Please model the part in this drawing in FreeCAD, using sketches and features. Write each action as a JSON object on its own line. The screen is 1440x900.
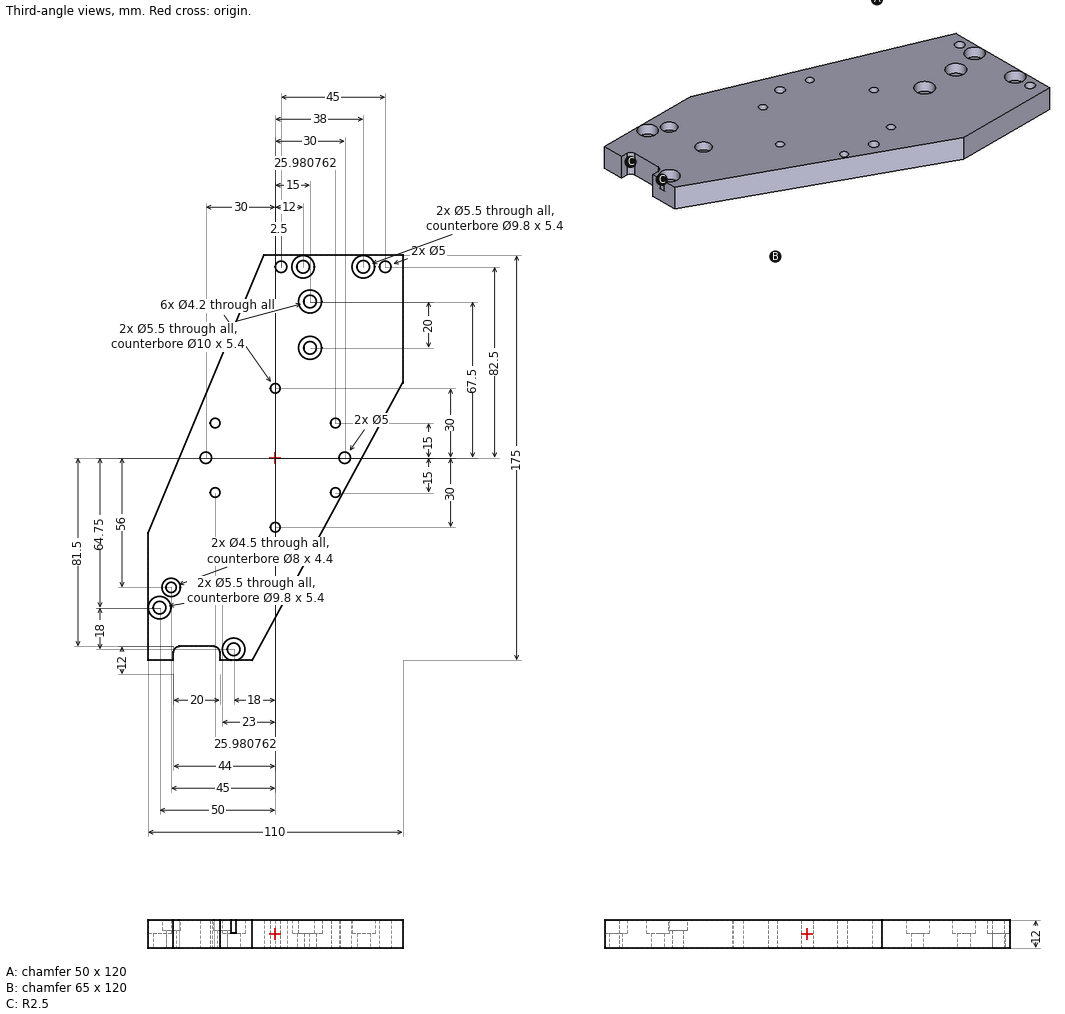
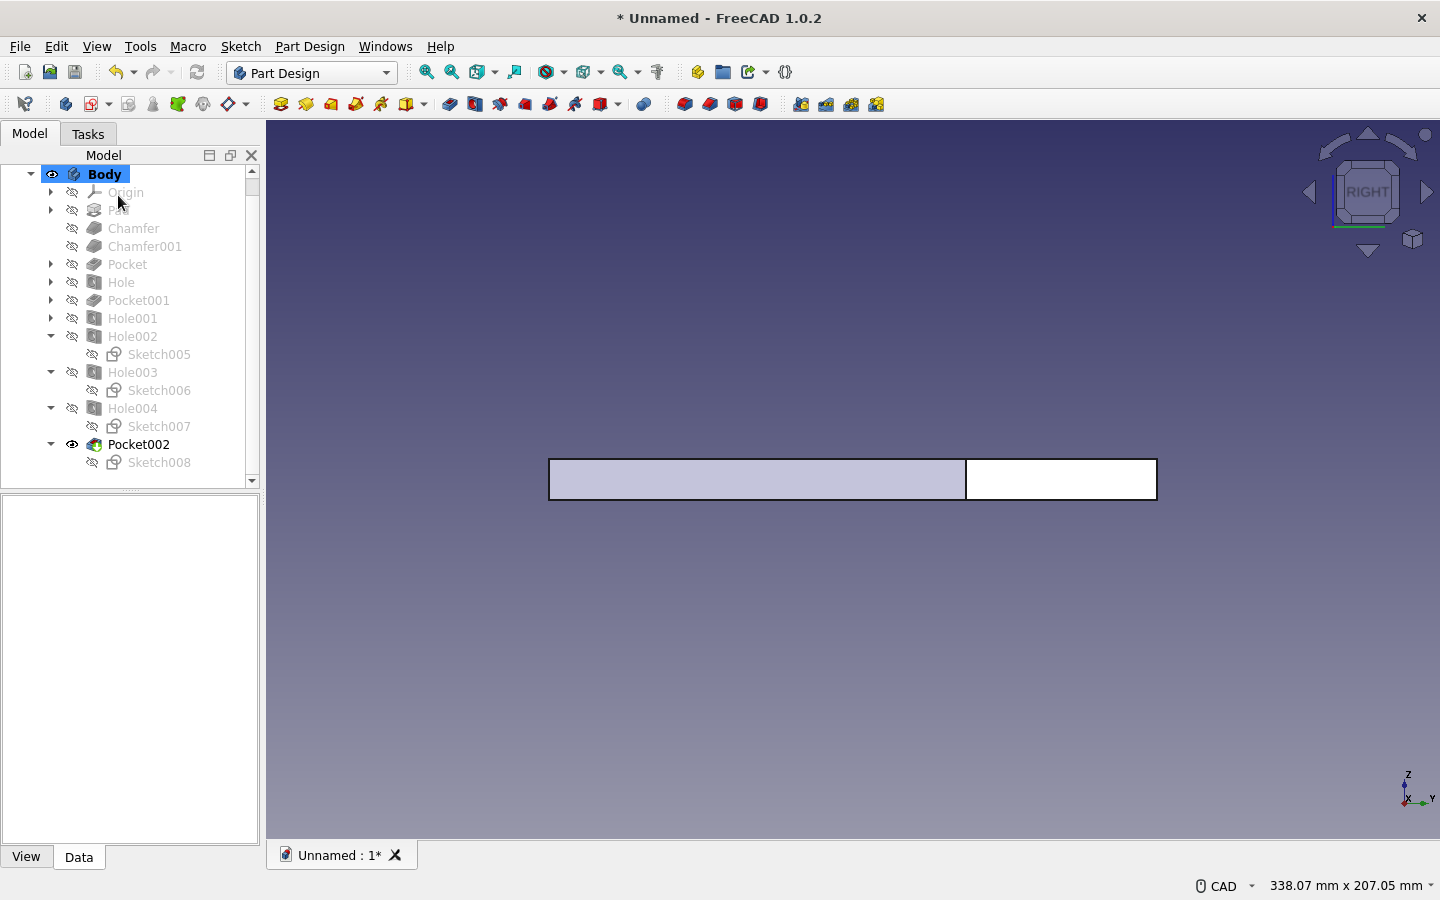
{"action": "key", "text": "5"}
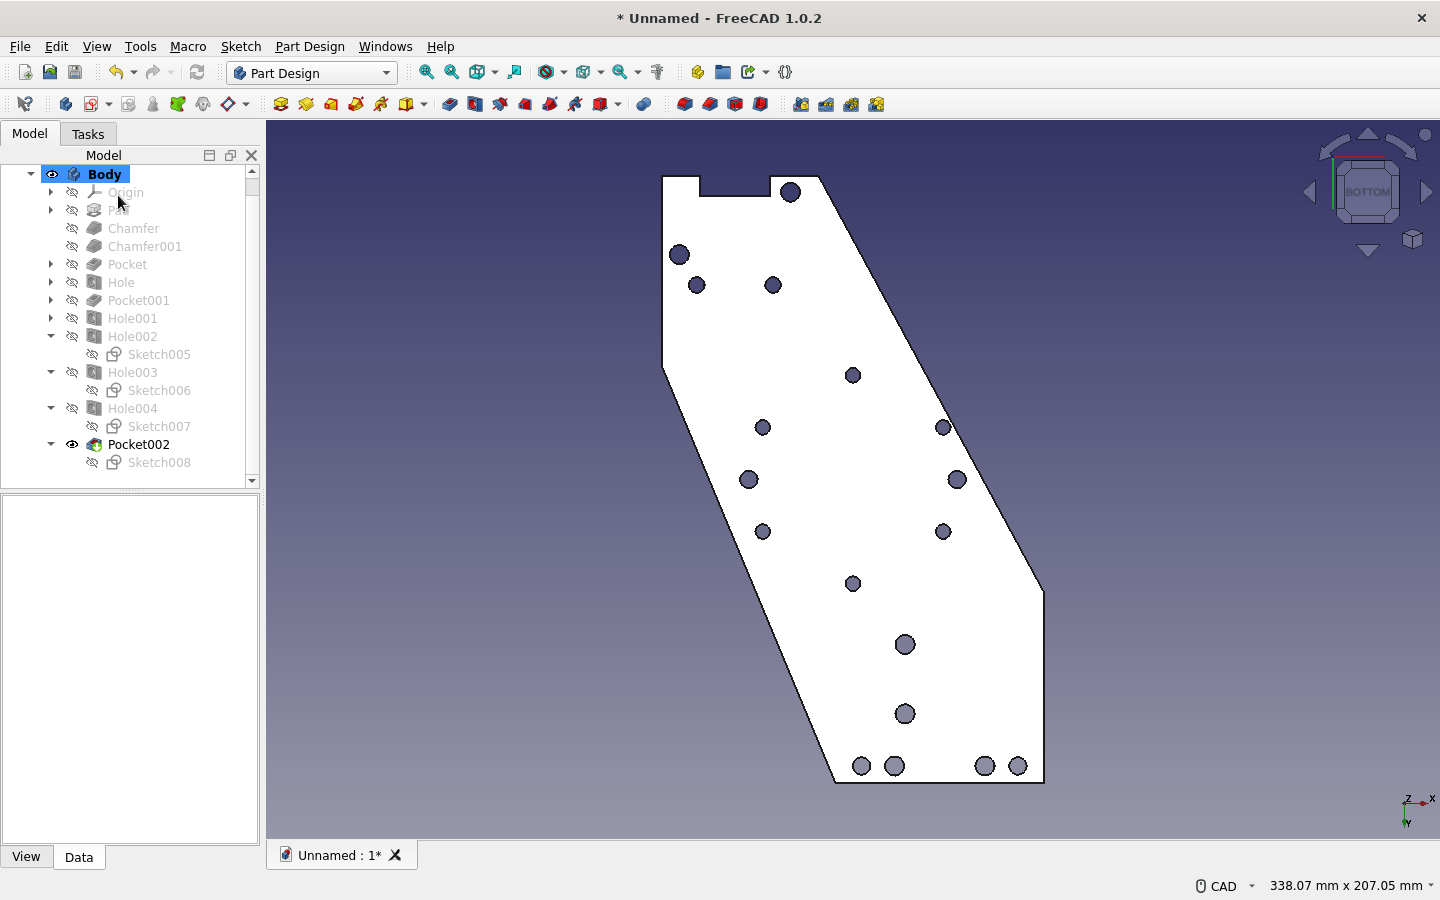
{"action": "key", "text": "4"}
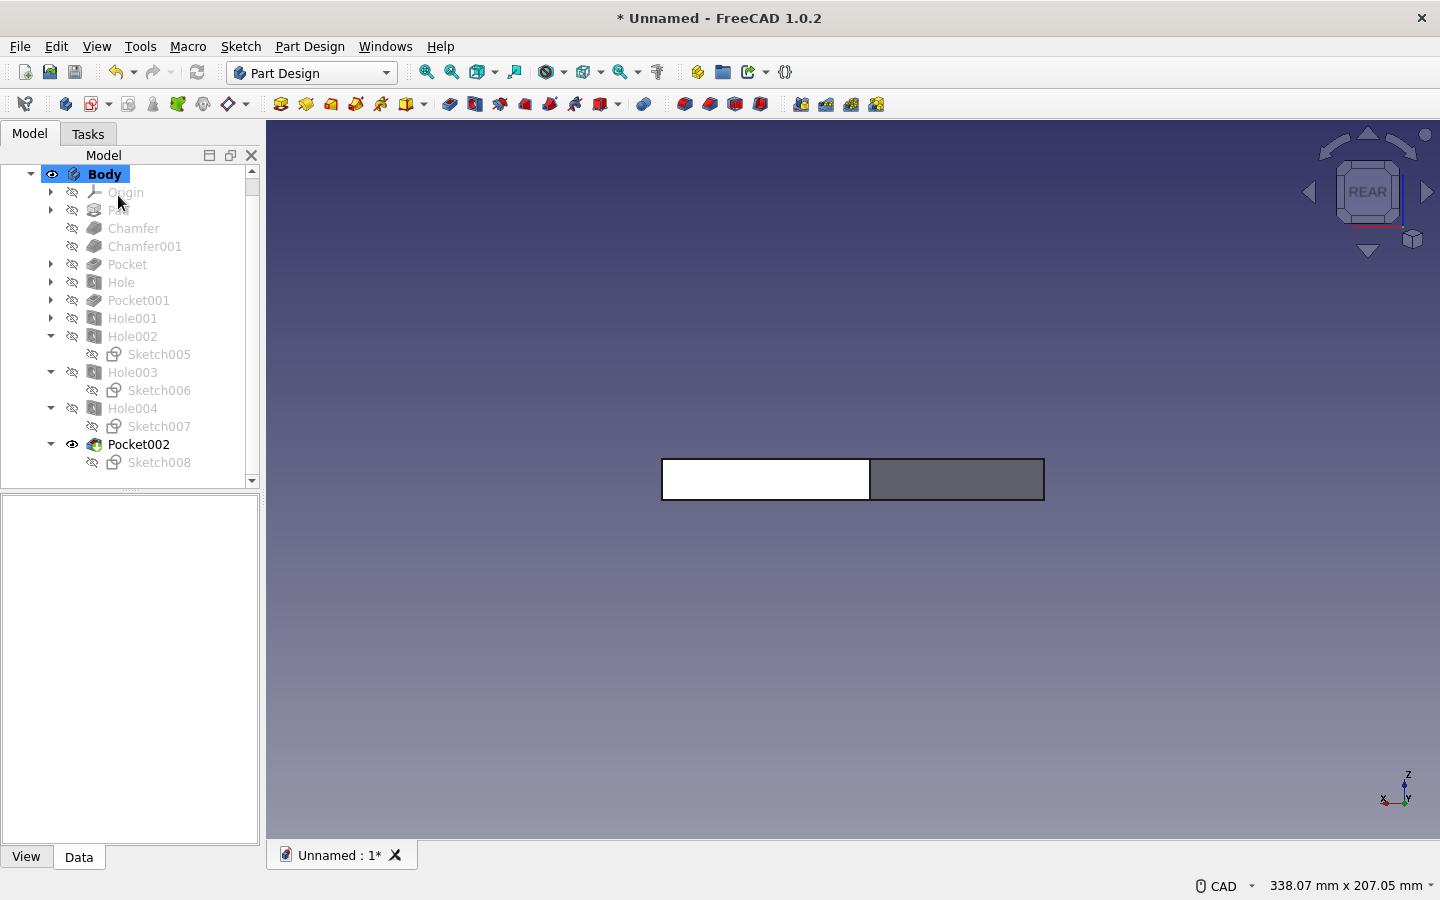
{"action": "key", "text": "v f"}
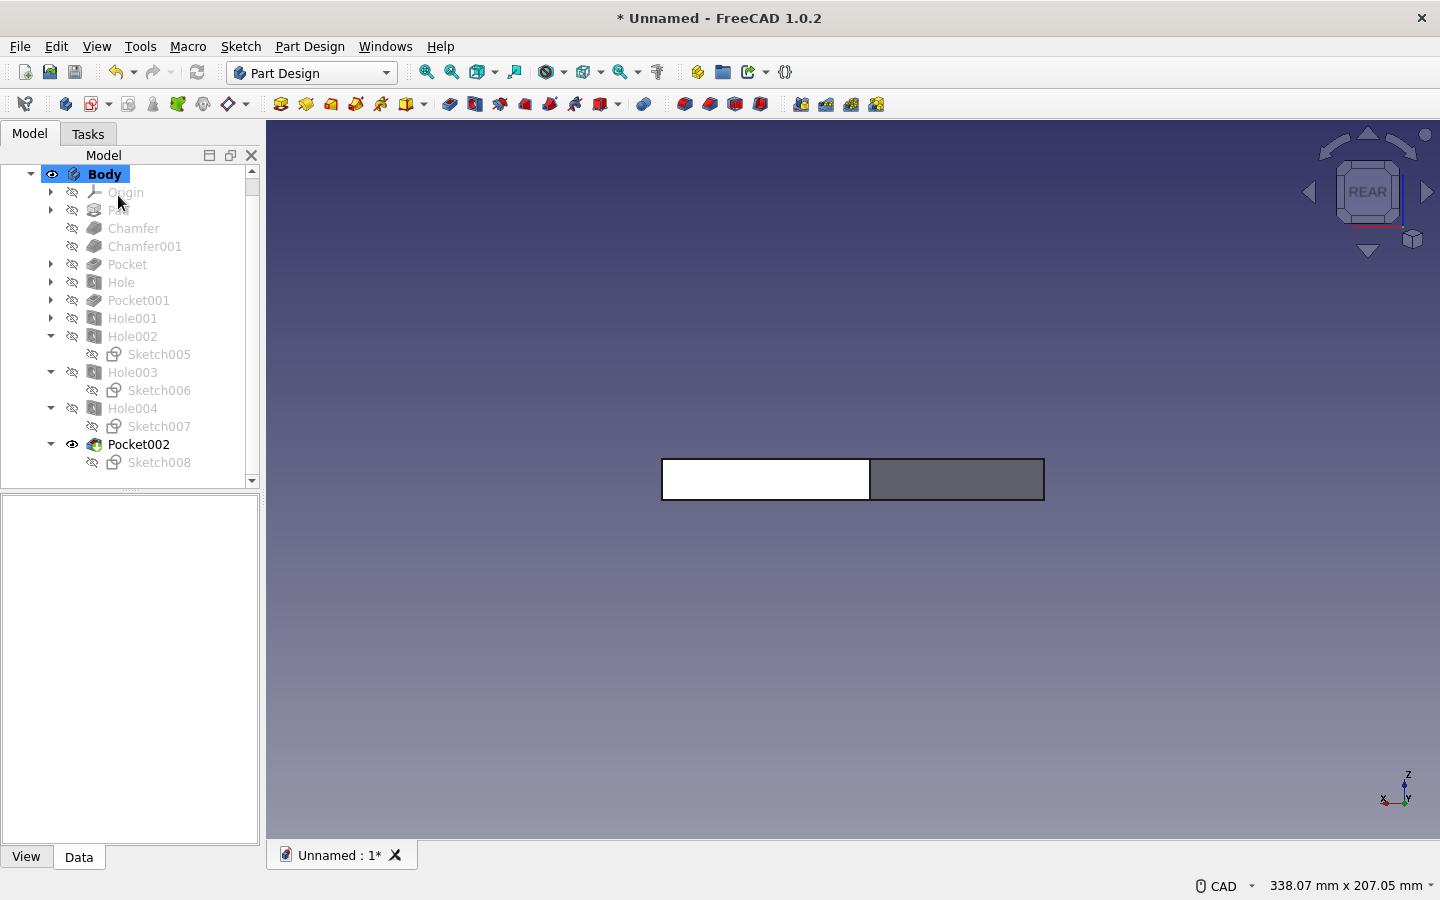
{"action": "key", "text": "6"}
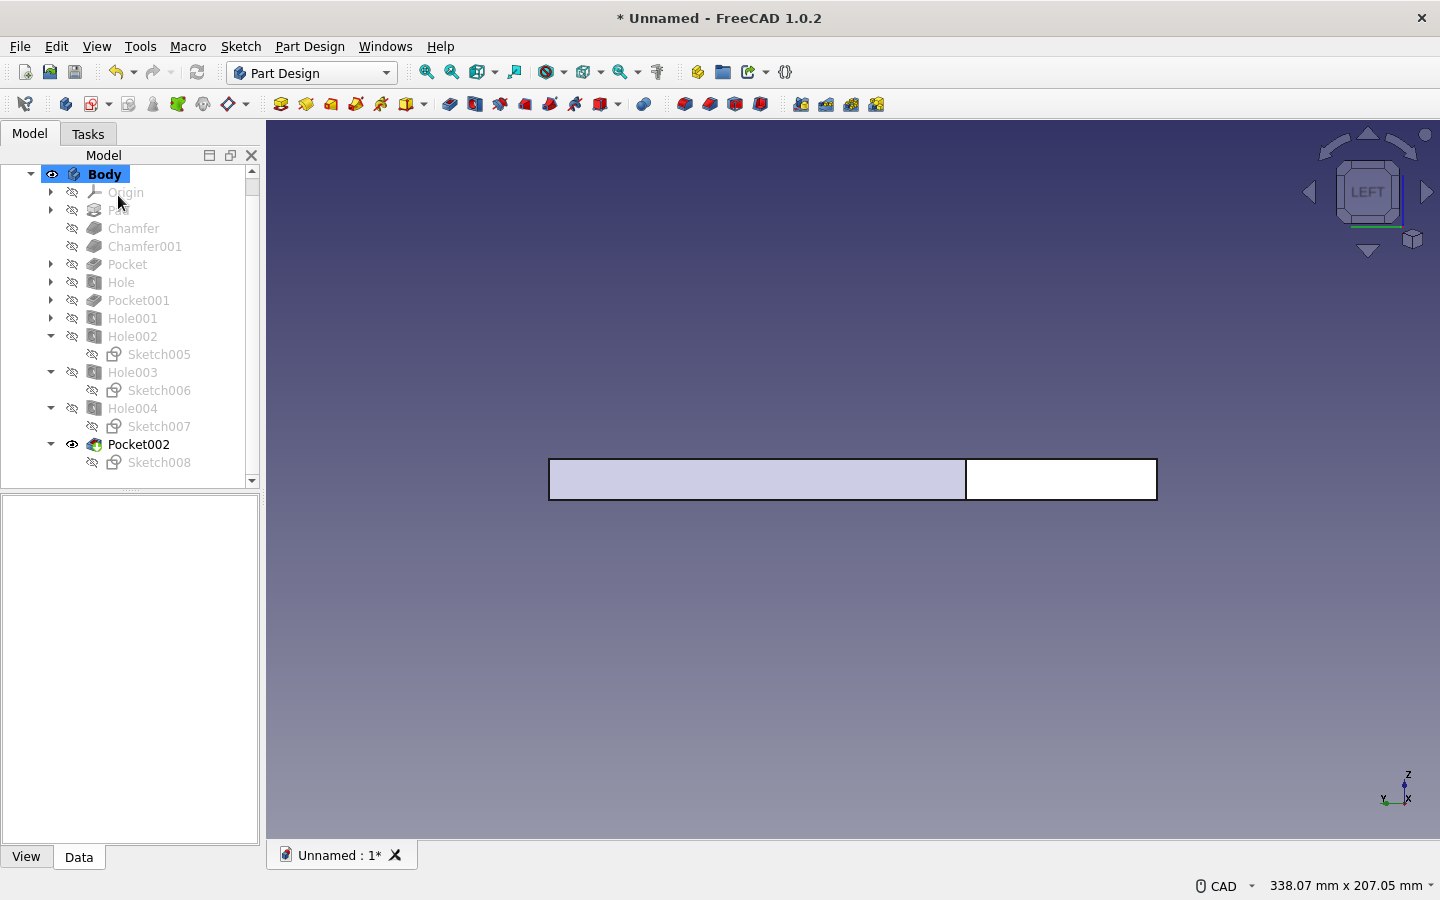
{"action": "key", "text": "v 3"}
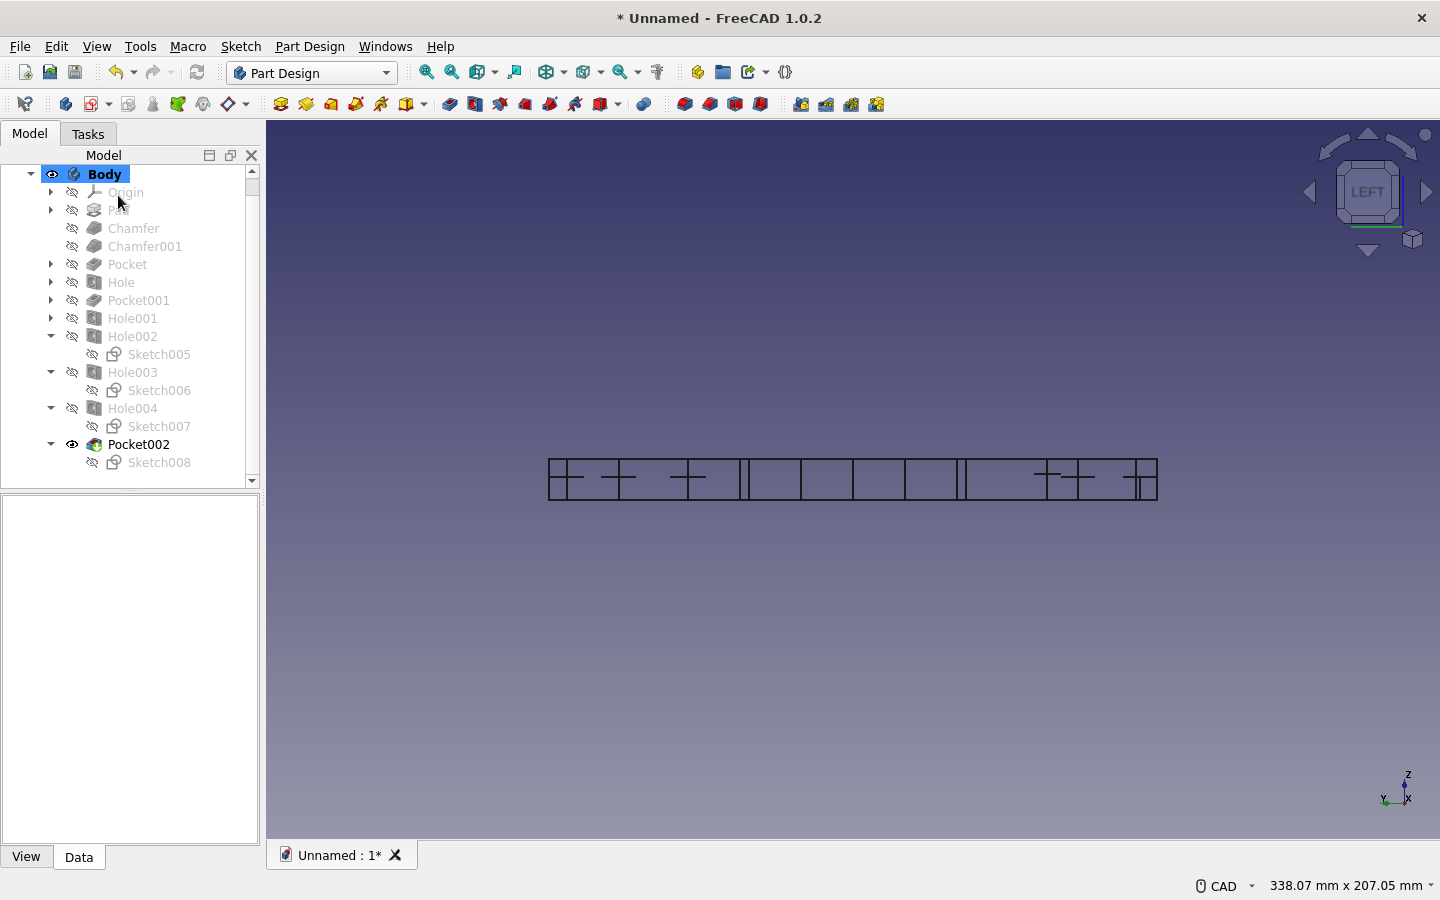
{"action": "key", "text": "0"}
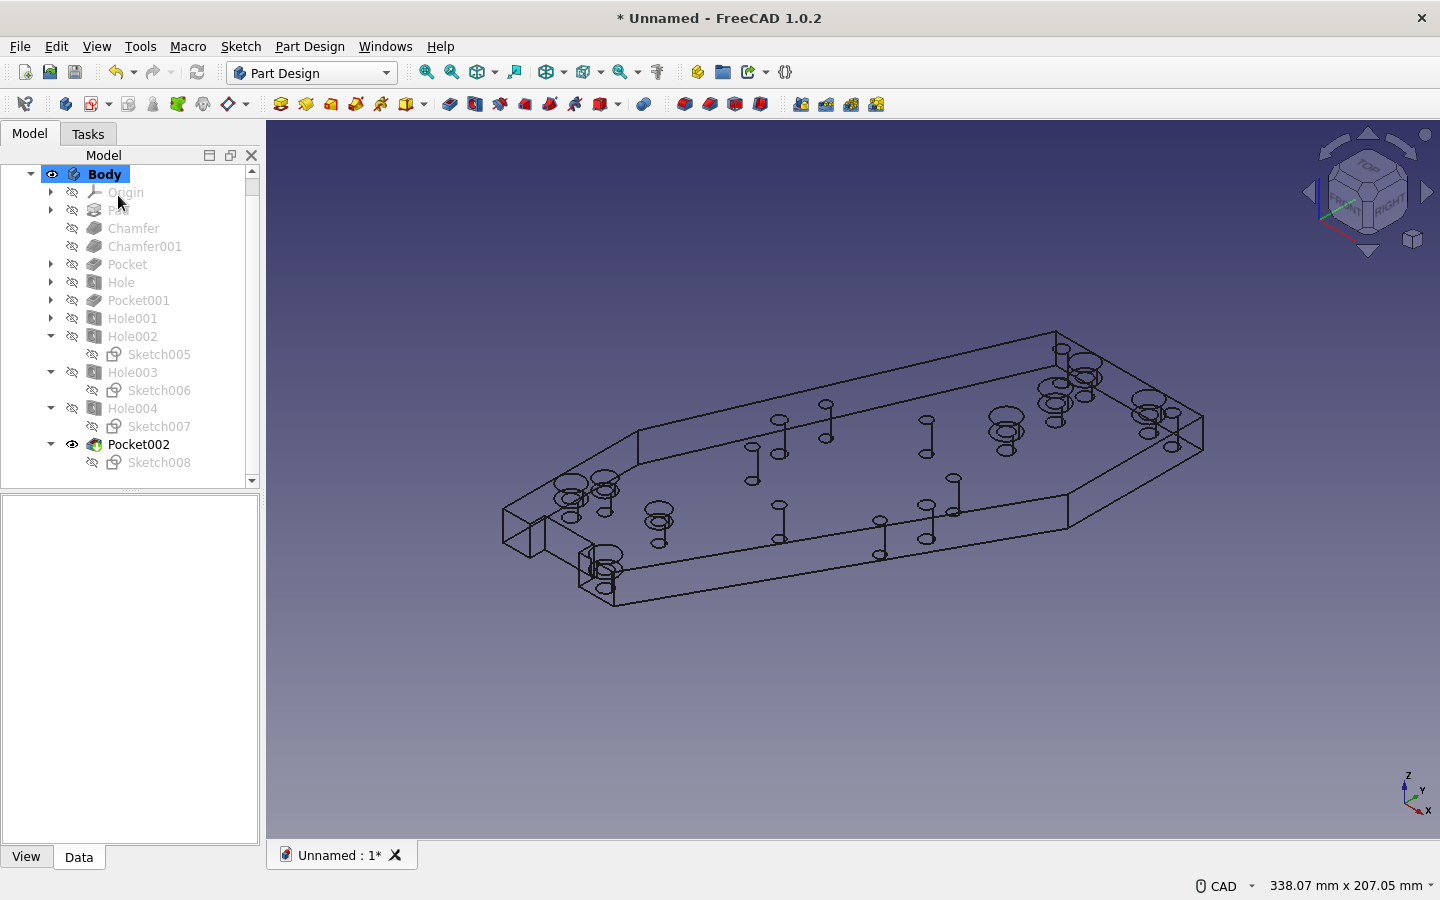
{"action": "left_click", "coordinate": [545, 532]}